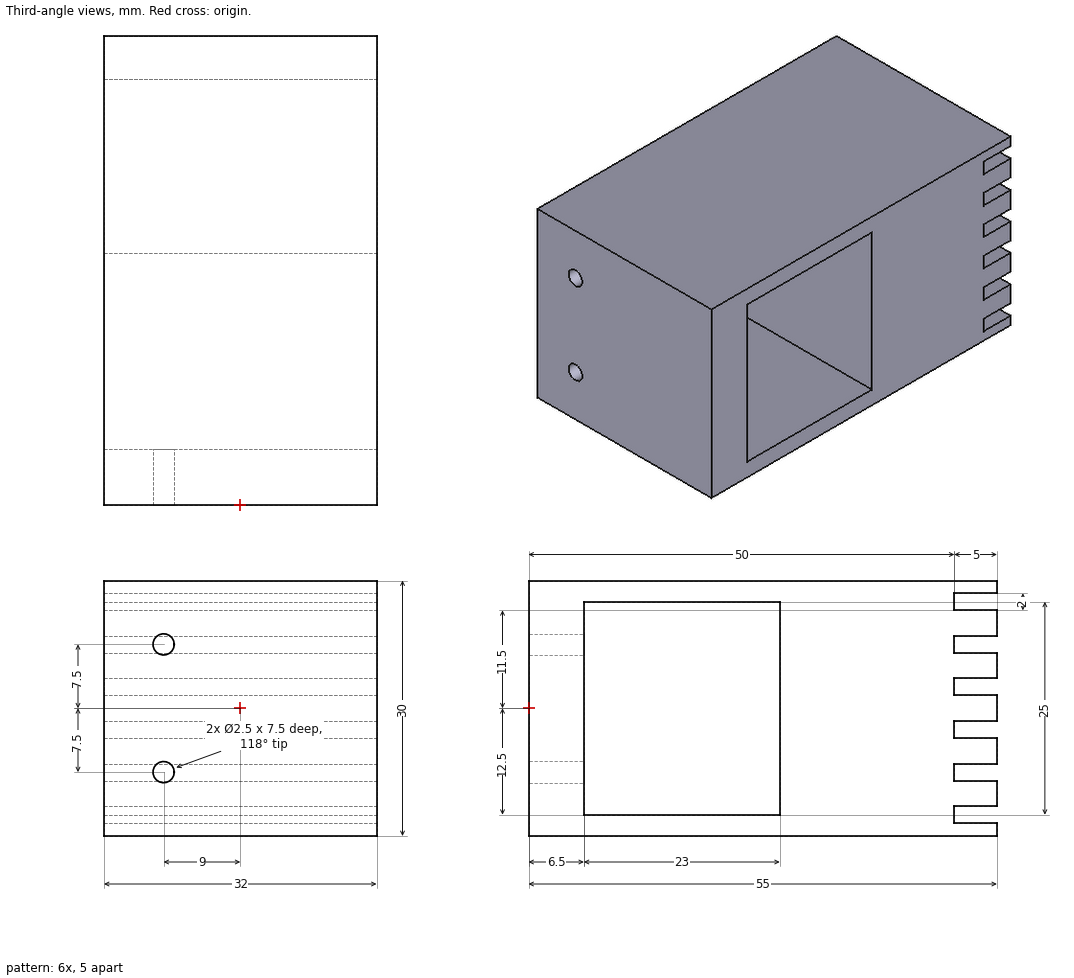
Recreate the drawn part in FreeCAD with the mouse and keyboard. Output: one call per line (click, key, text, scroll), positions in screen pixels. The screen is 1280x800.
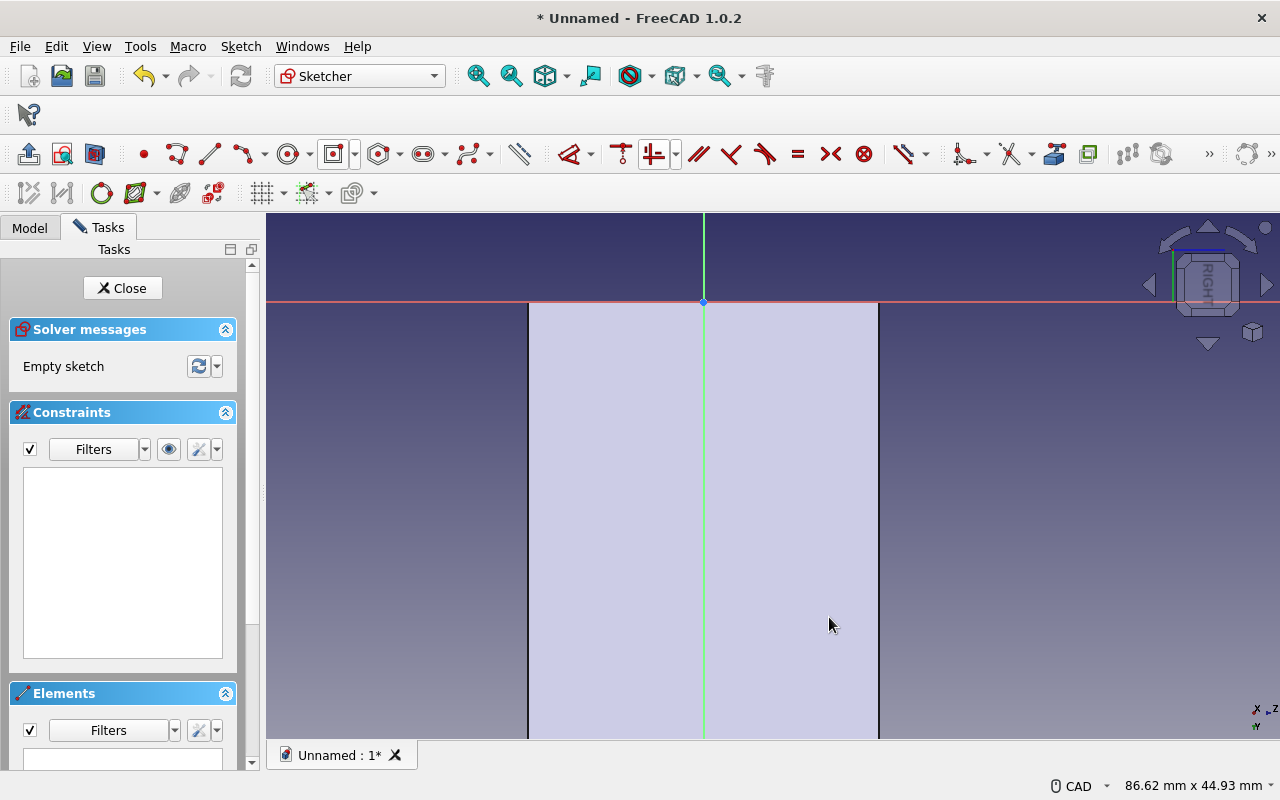
click(354, 154)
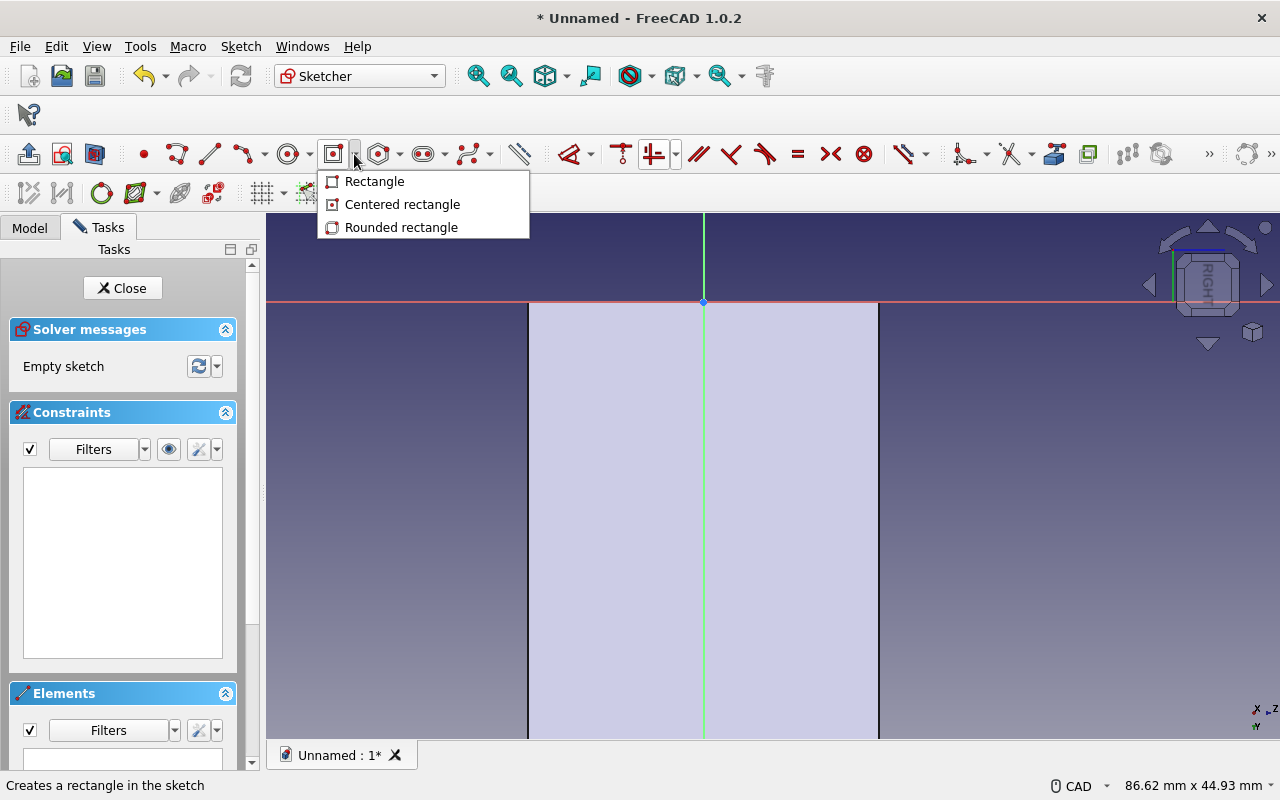
click(424, 182)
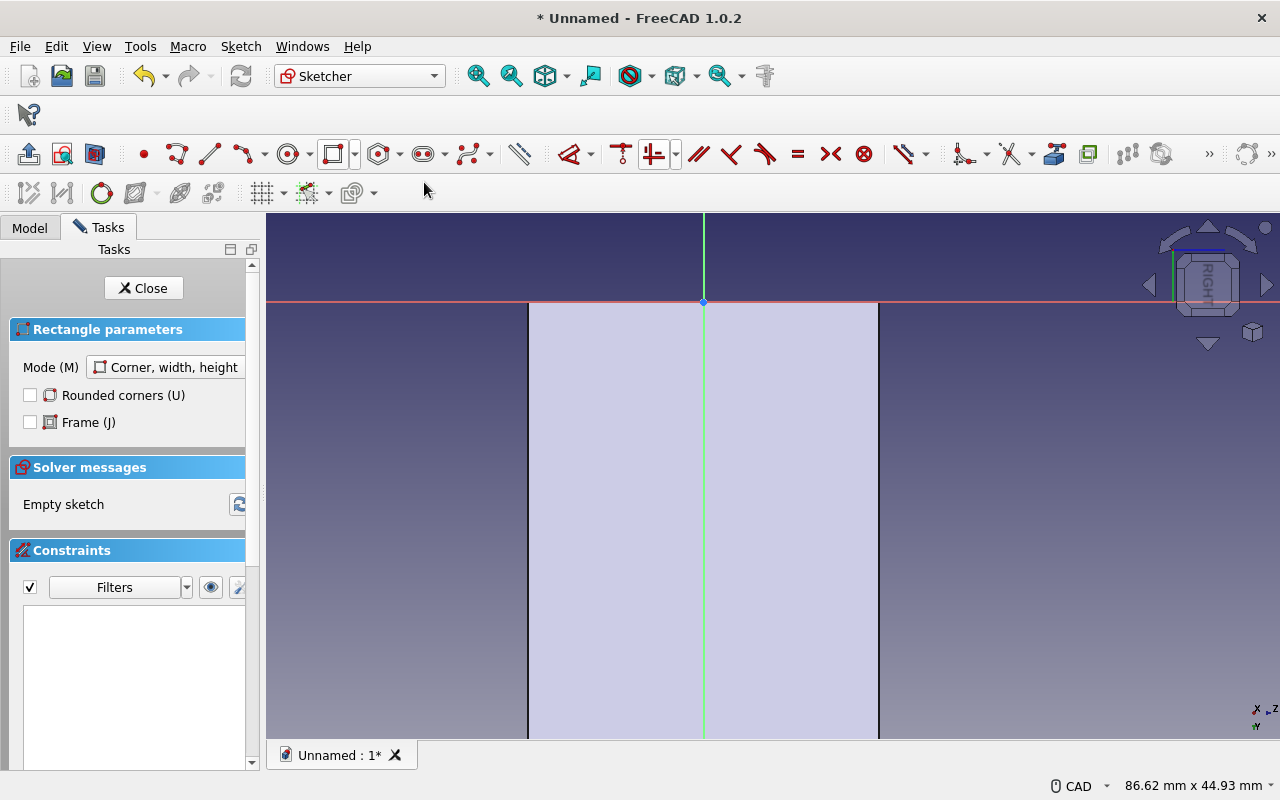
click(557, 378)
click(850, 648)
key(Escape)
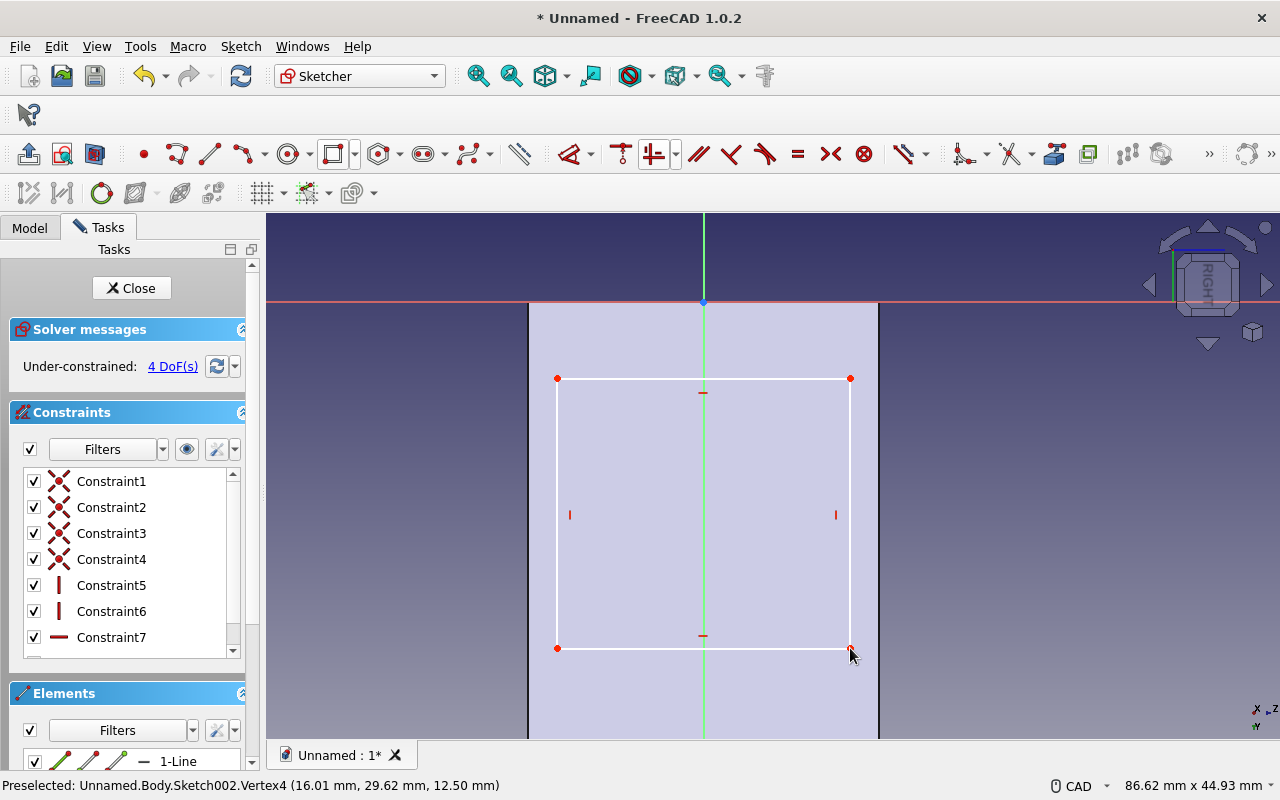
click(568, 154)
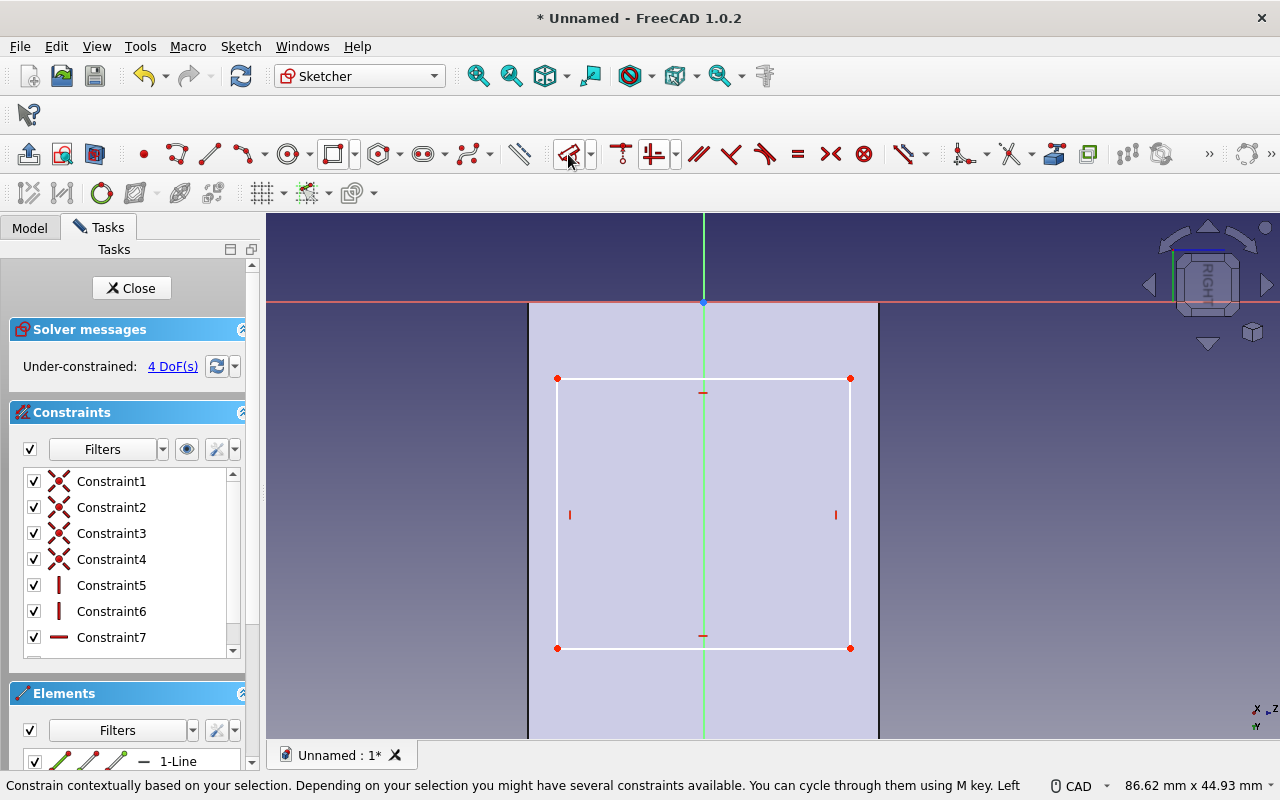
click(557, 460)
click(523, 514)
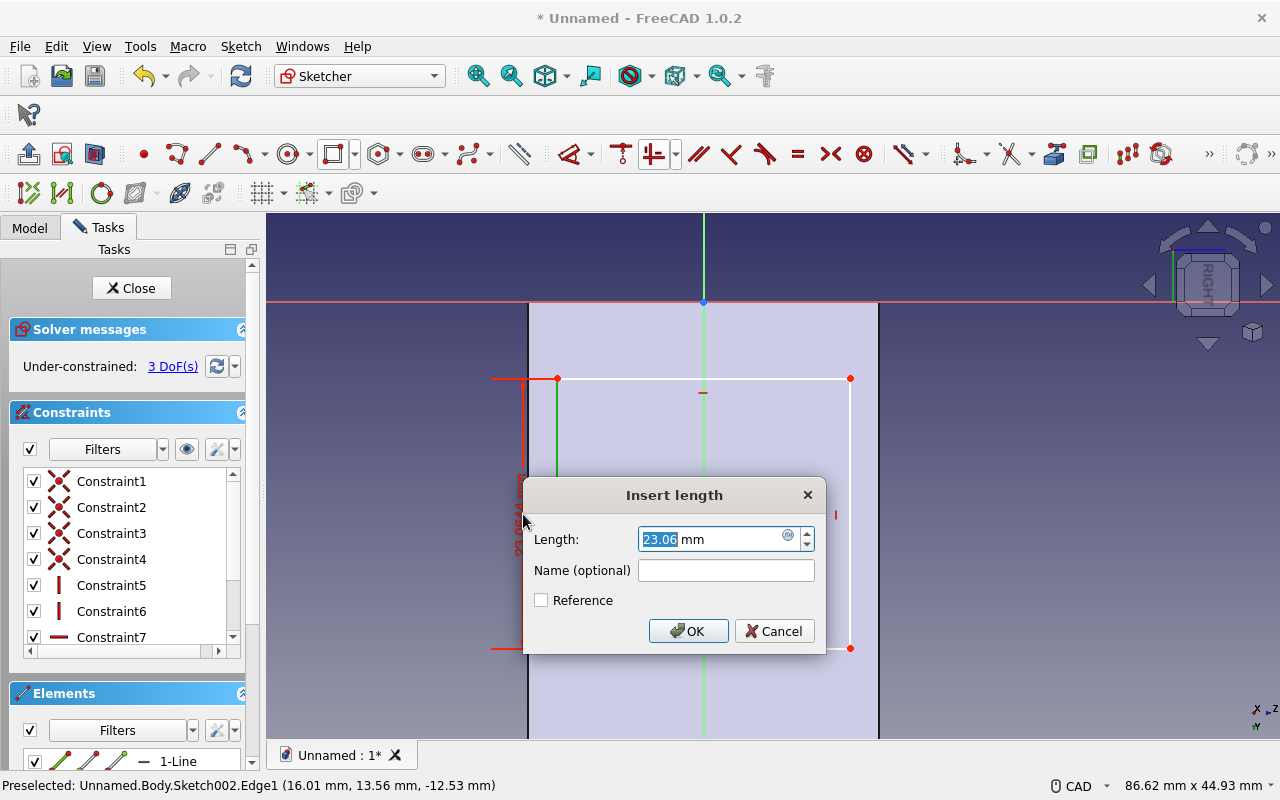
text(23)
key(Return)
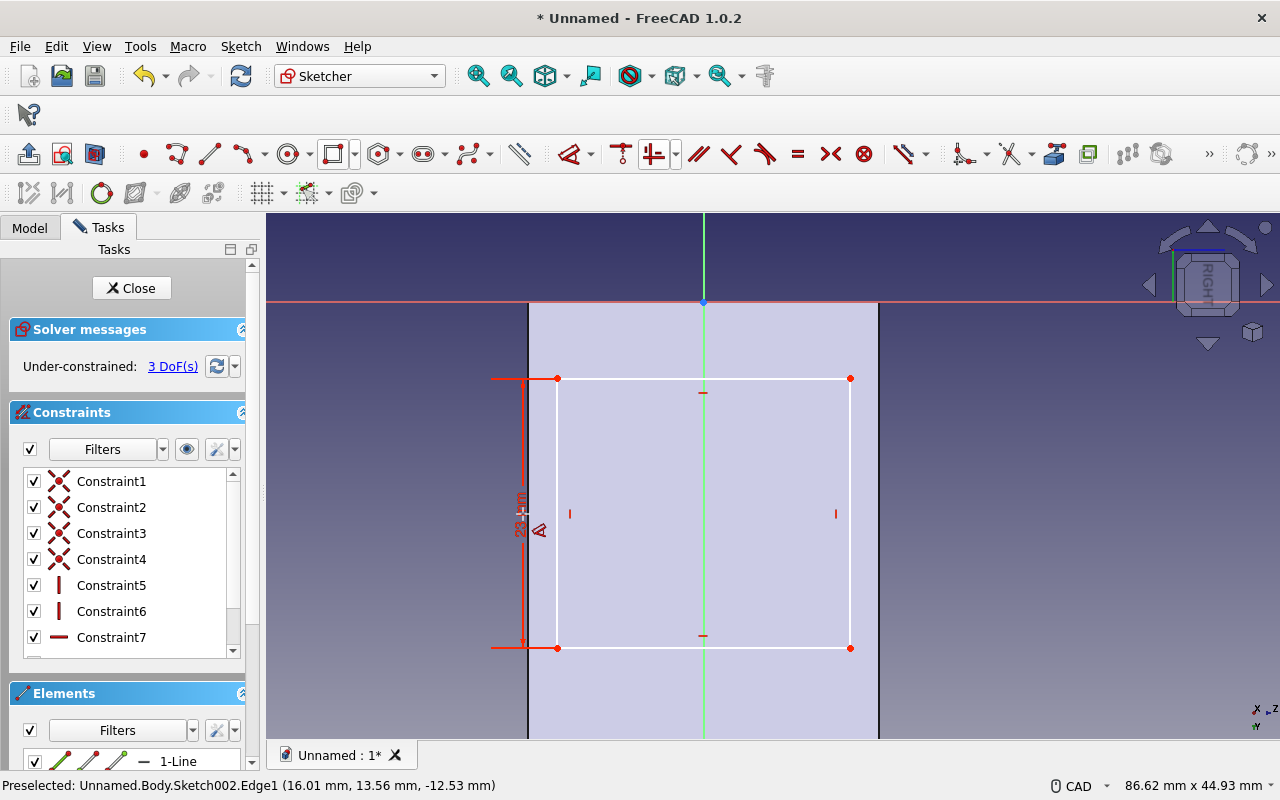
click(645, 648)
click(636, 682)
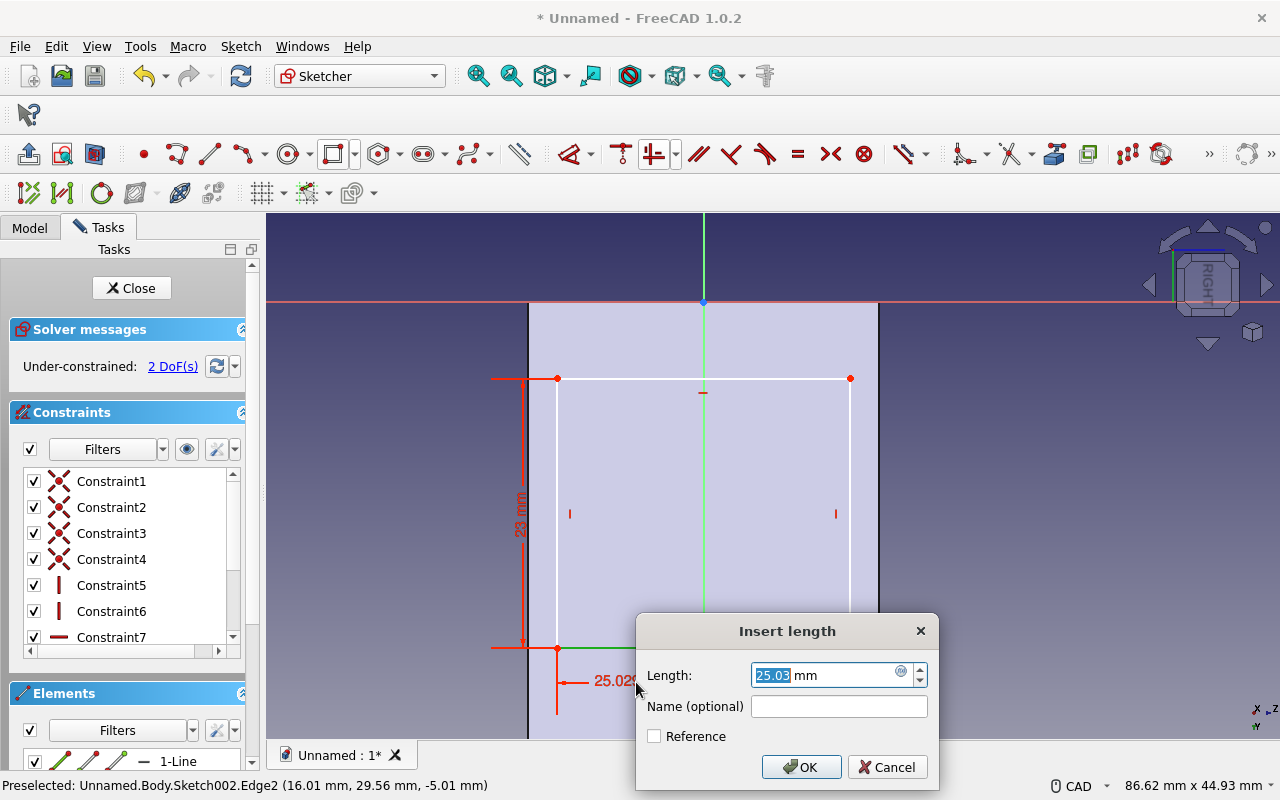
text(25)
key(Return)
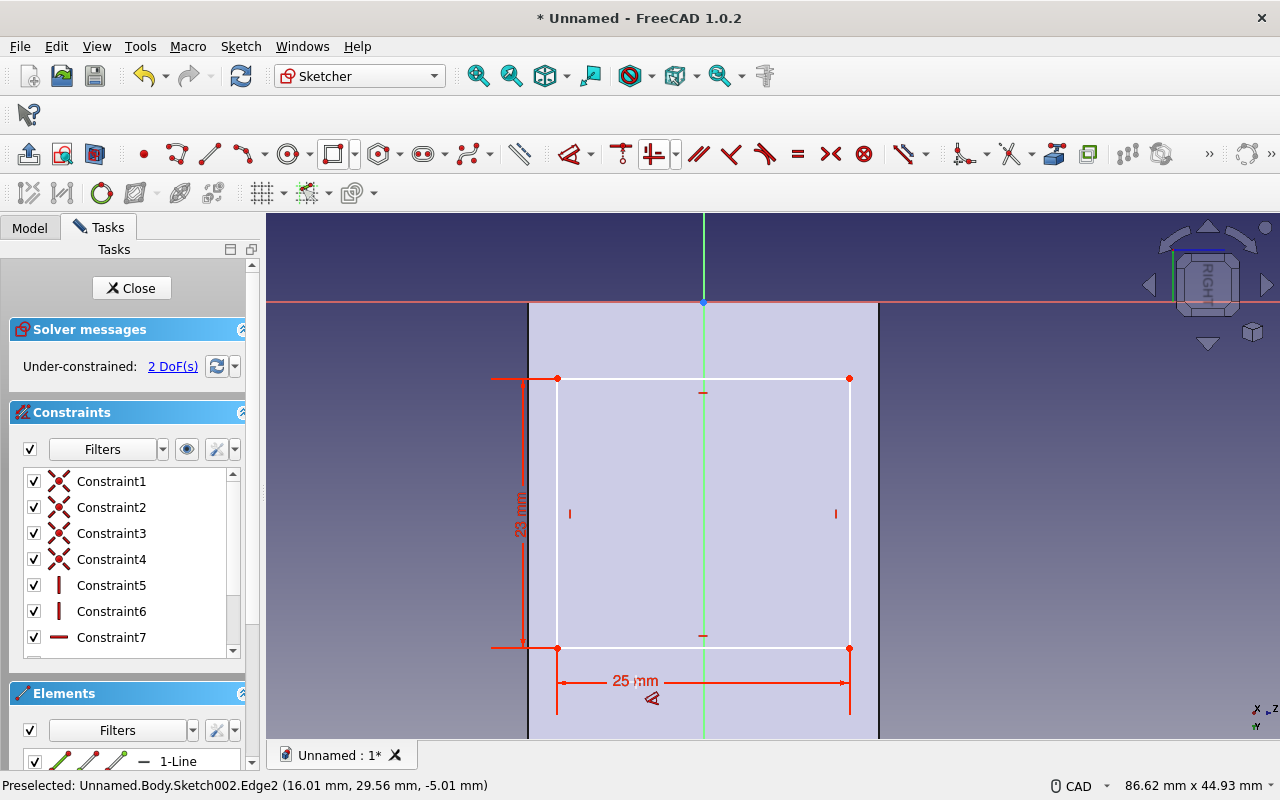
click(557, 379)
click(523, 341)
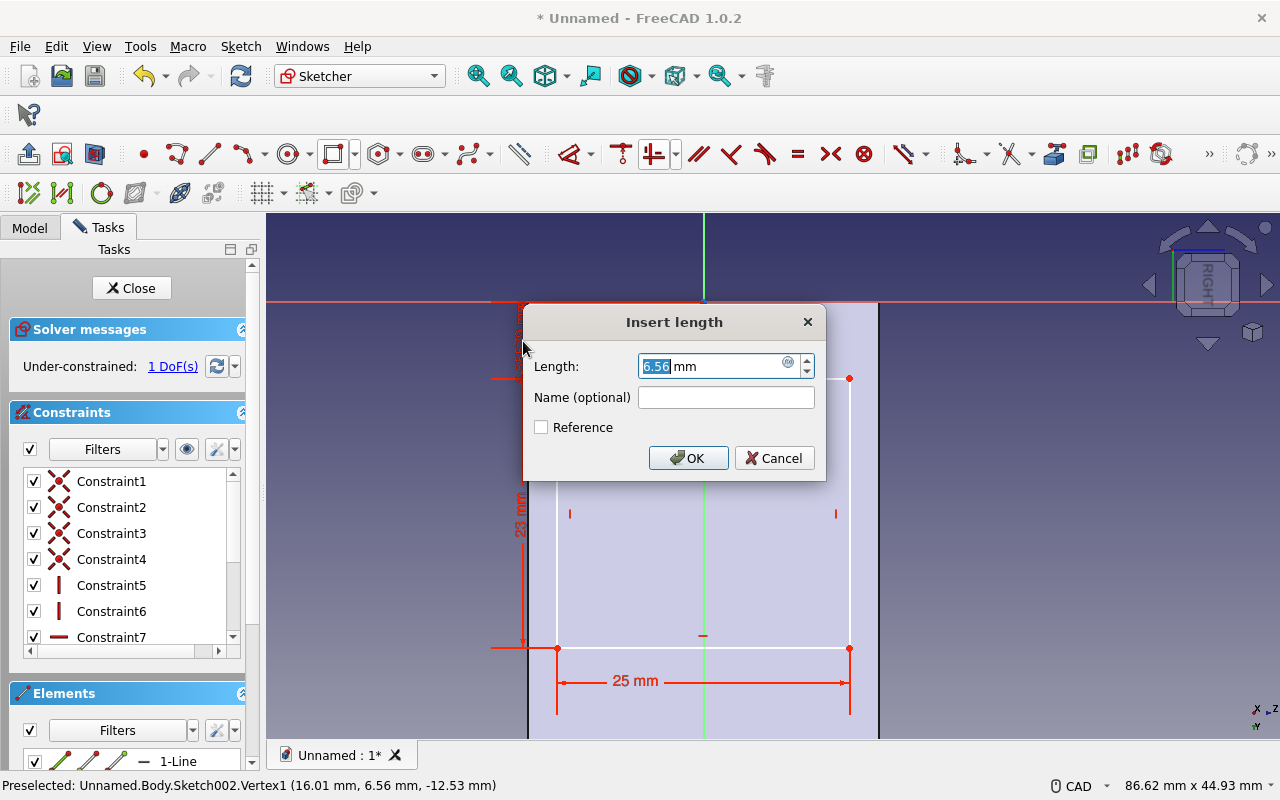
text(6.5)
key(Return)